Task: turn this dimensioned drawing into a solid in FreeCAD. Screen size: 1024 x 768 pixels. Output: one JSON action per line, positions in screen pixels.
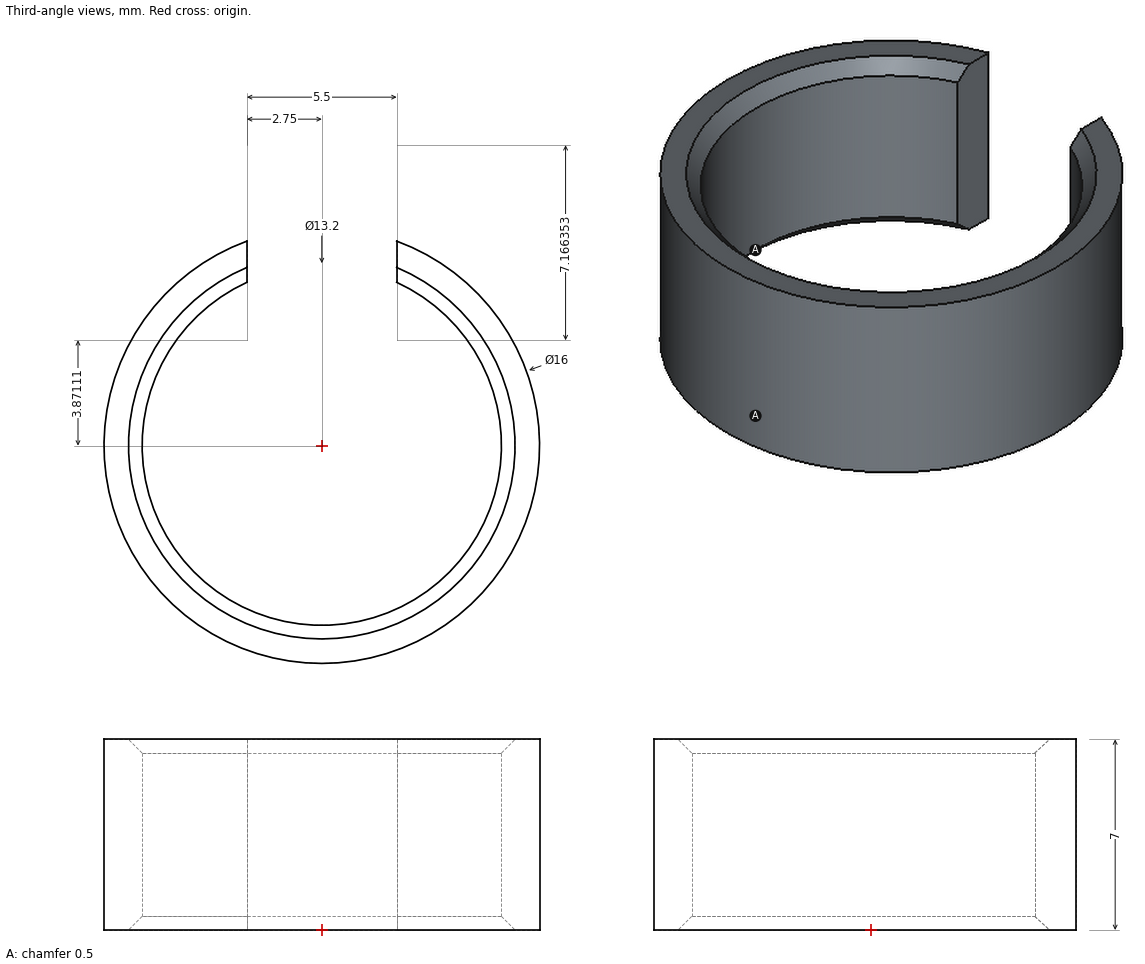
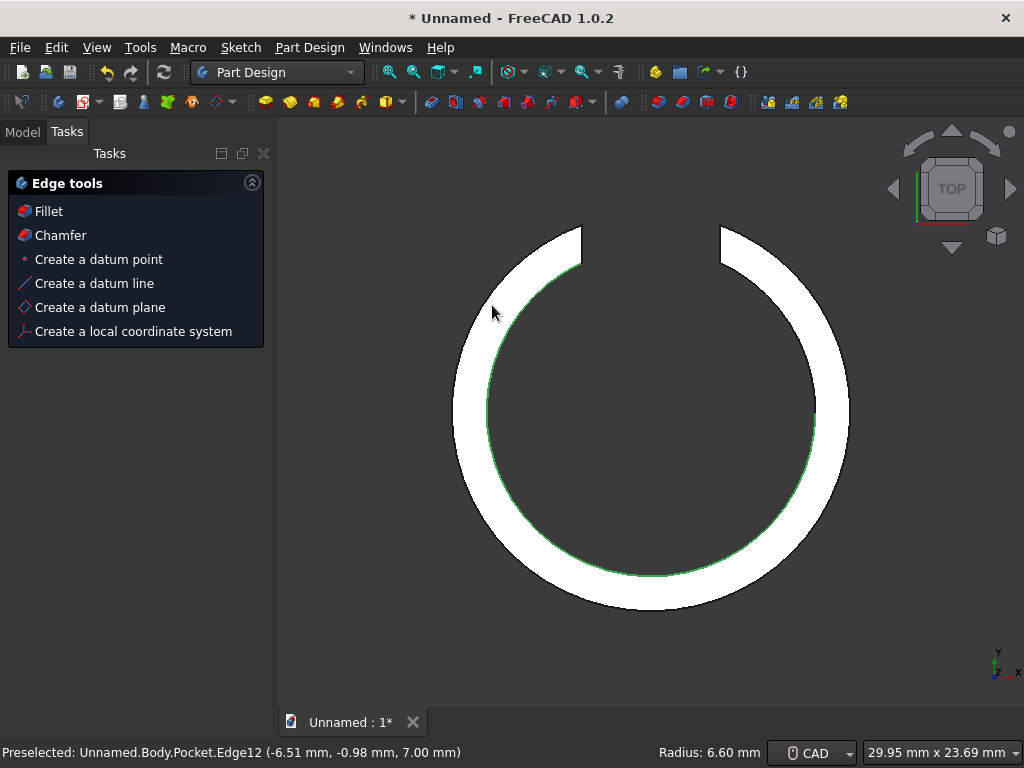
{"action": "key", "text": "1"}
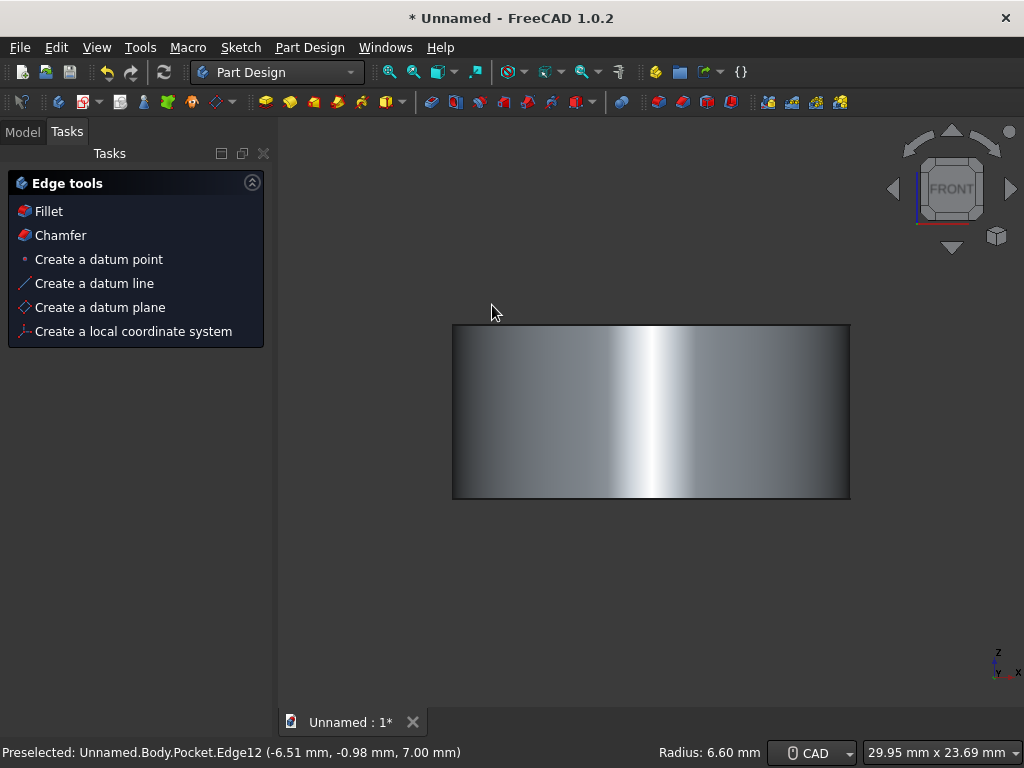
{"action": "key", "text": "3"}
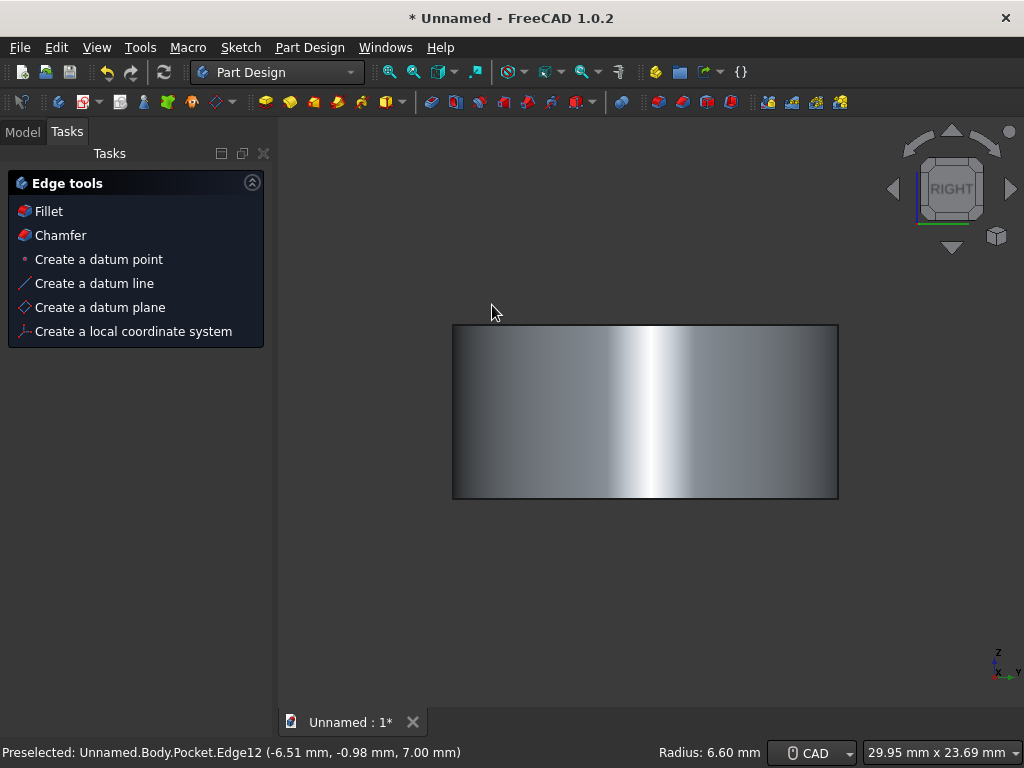
{"action": "key", "text": "5"}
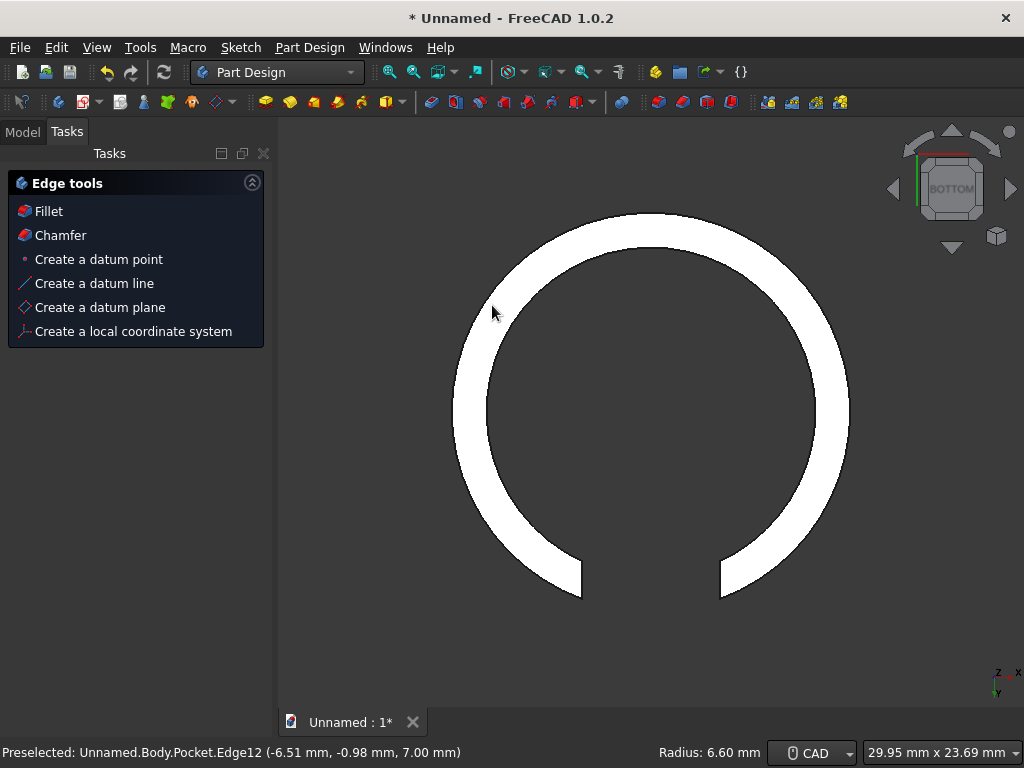
{"action": "left_click", "coordinate": [513, 322], "text": "ctrl"}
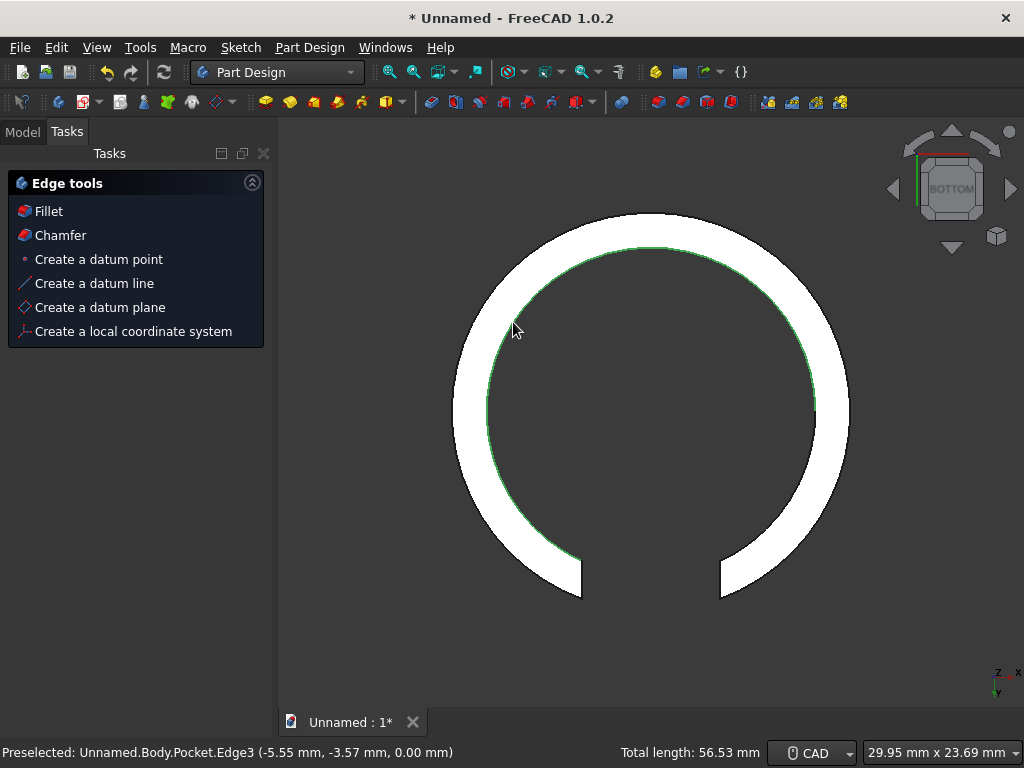
{"action": "left_click", "coordinate": [684, 102]}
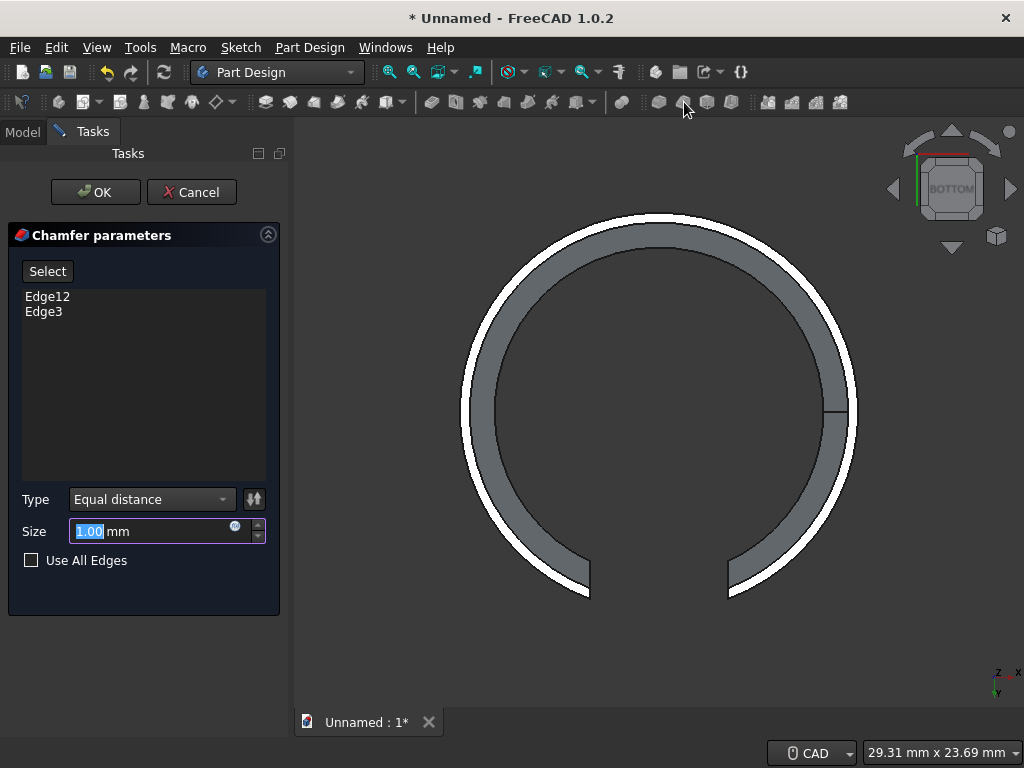
{"action": "type", "text": "0.5"}
{"action": "key", "text": "Tab"}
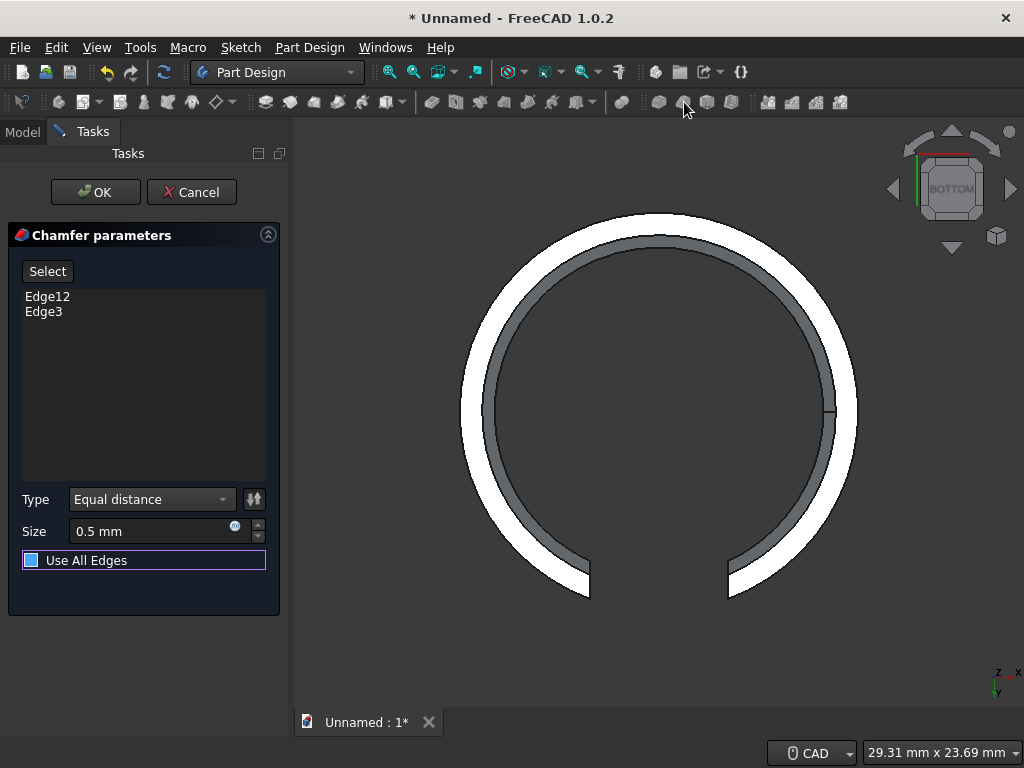
{"action": "left_click", "coordinate": [96, 192]}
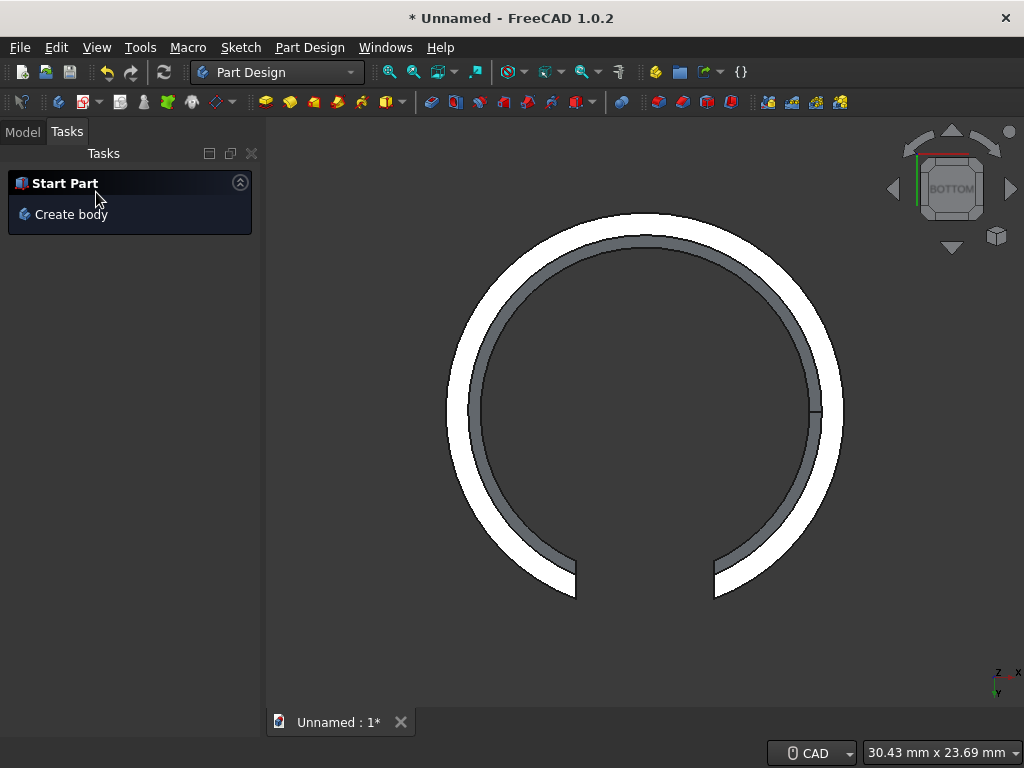
{"action": "key", "text": "0"}